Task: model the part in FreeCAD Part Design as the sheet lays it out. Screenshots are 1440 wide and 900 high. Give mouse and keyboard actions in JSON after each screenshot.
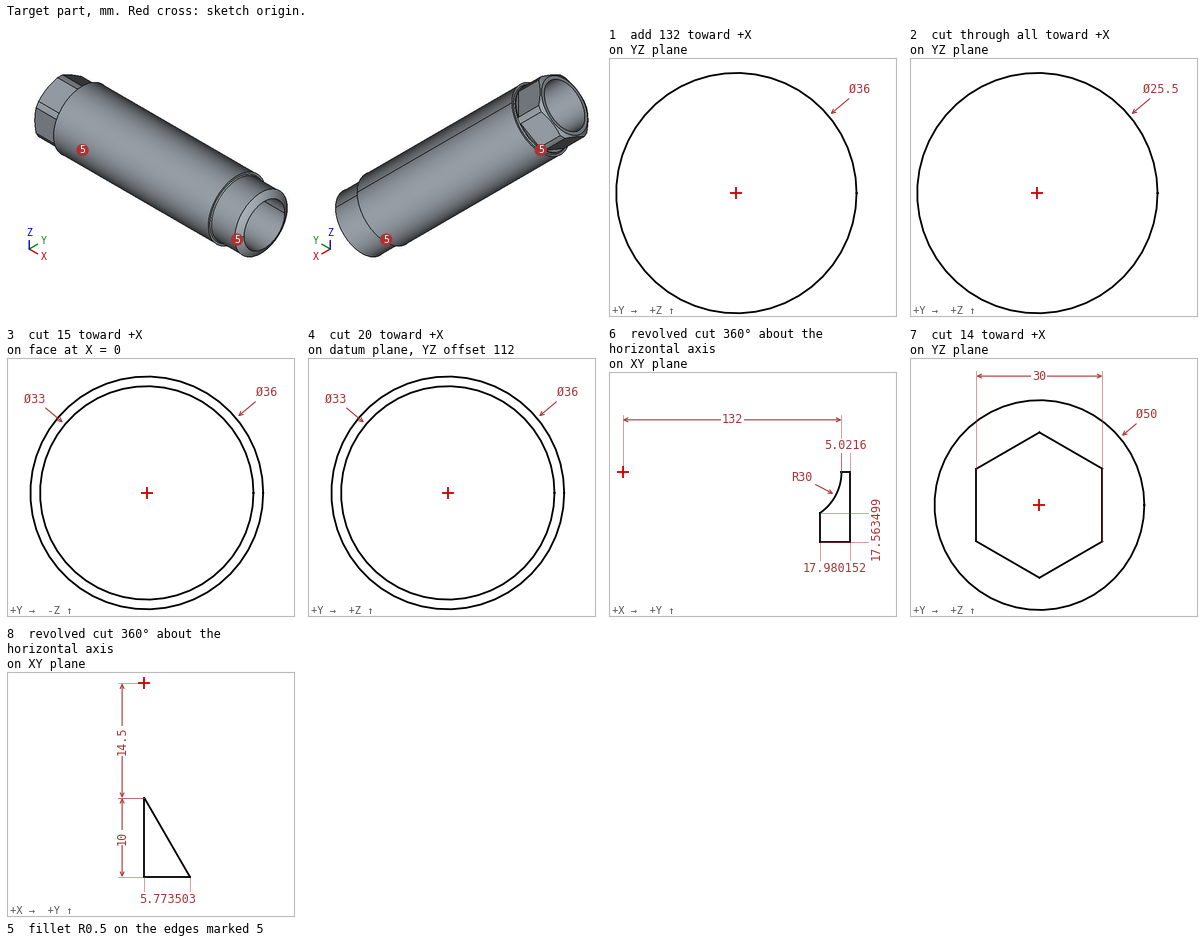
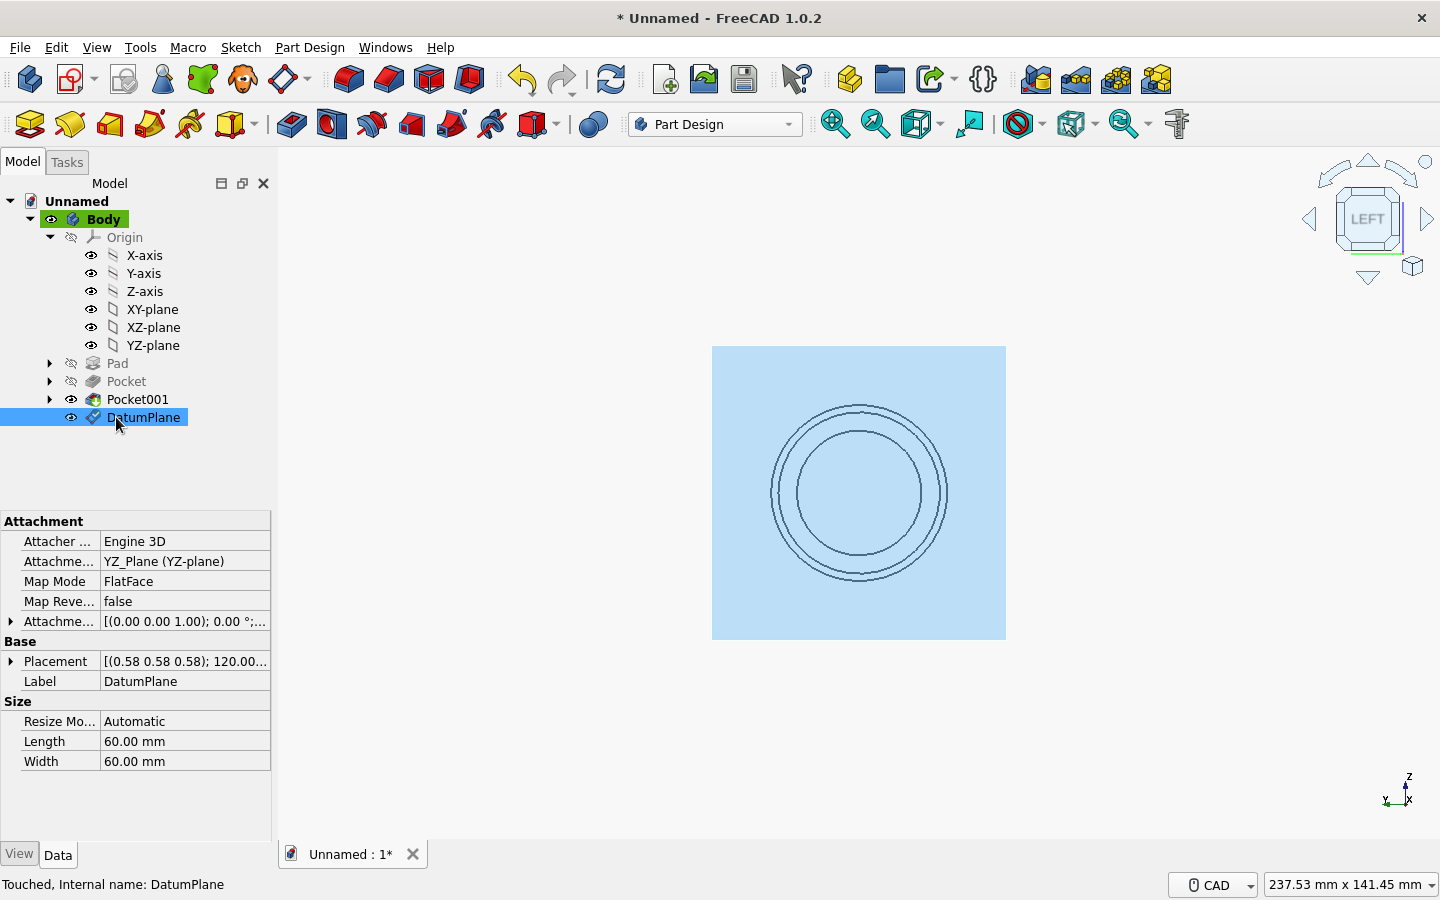
{"action": "left_click", "coordinate": [70, 80]}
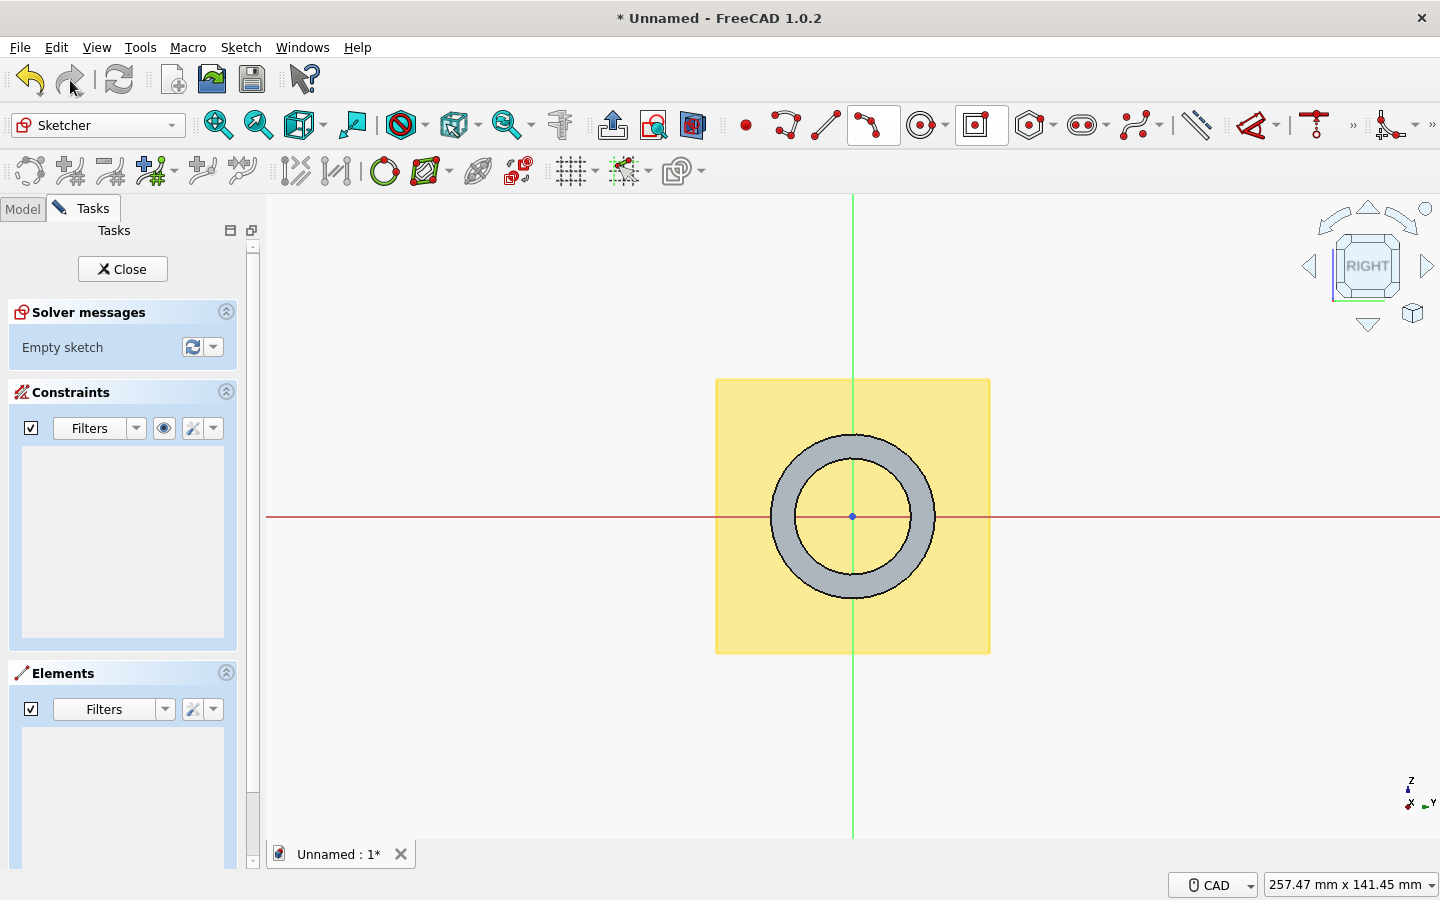
{"action": "key", "text": "q s"}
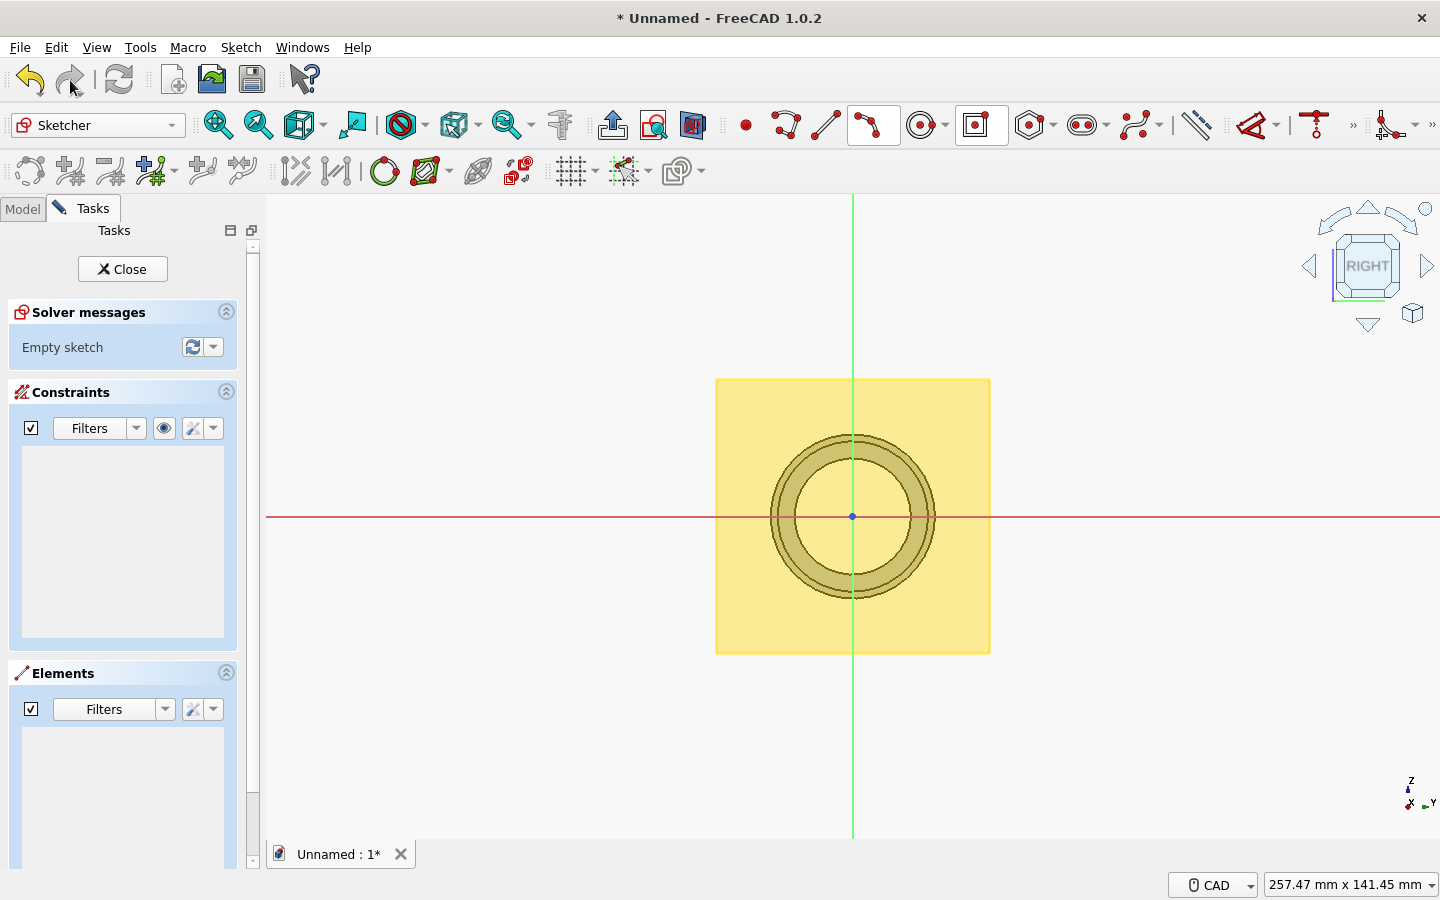
{"action": "scroll", "coordinate": [893, 516], "scroll_direction": "up", "scroll_amount": 5}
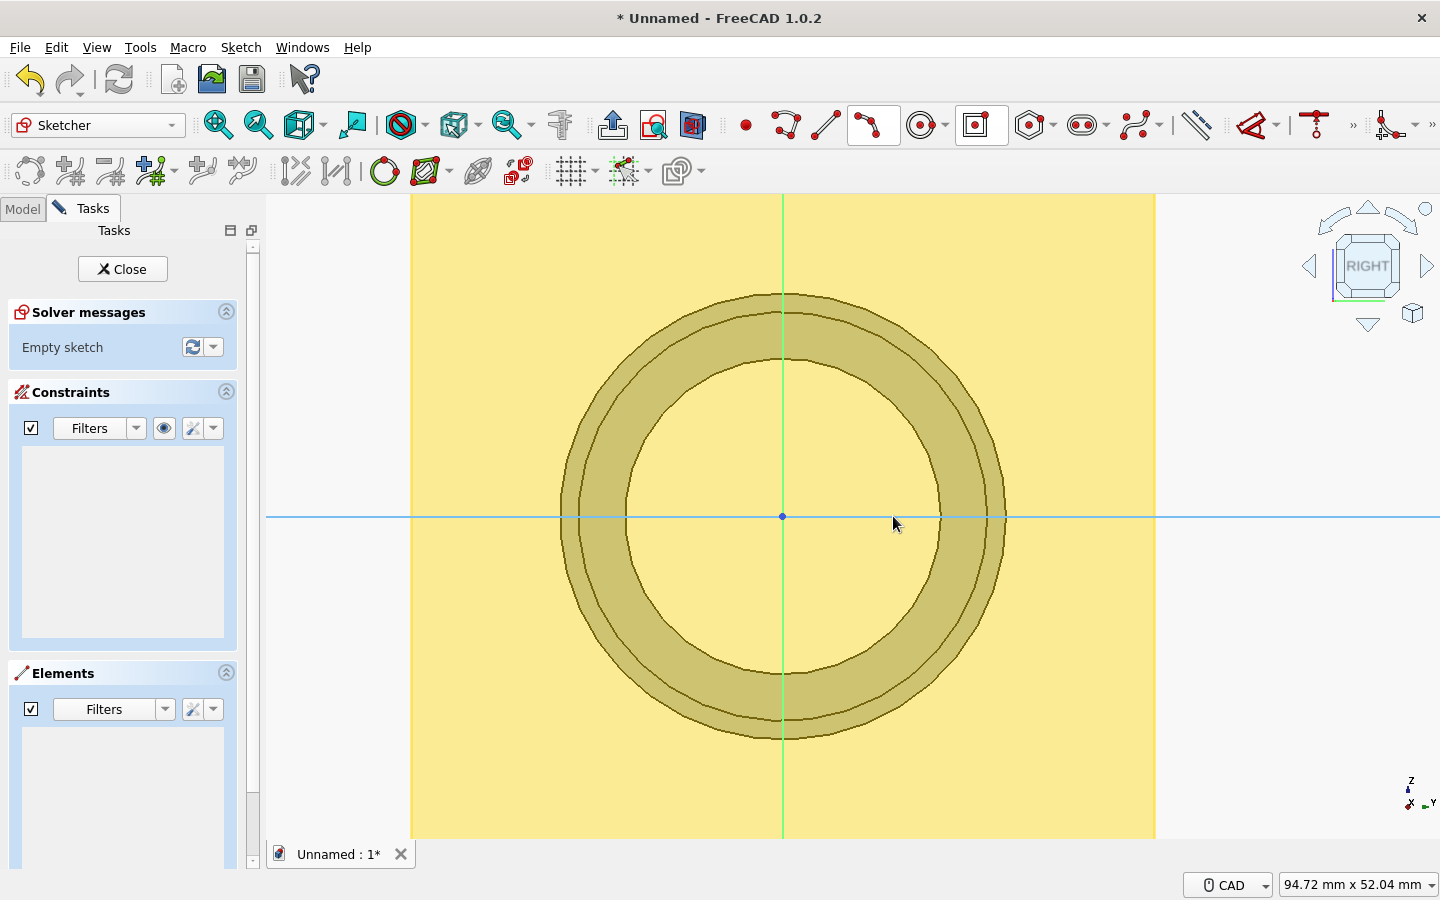
{"action": "left_click", "coordinate": [922, 126]}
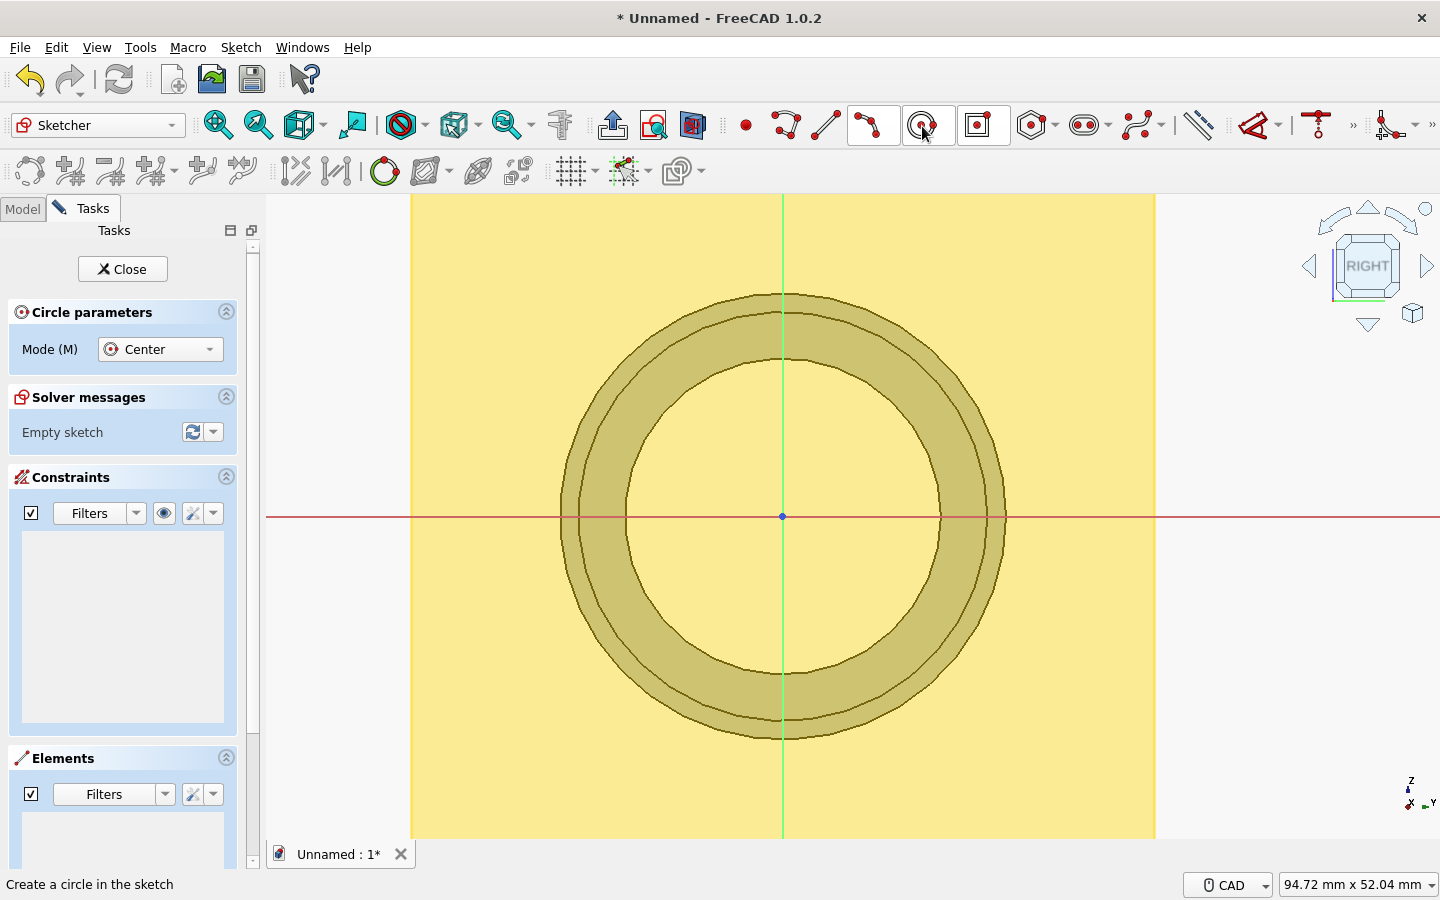
{"action": "left_click", "coordinate": [783, 516]}
{"action": "mouse_move", "coordinate": [941, 359]}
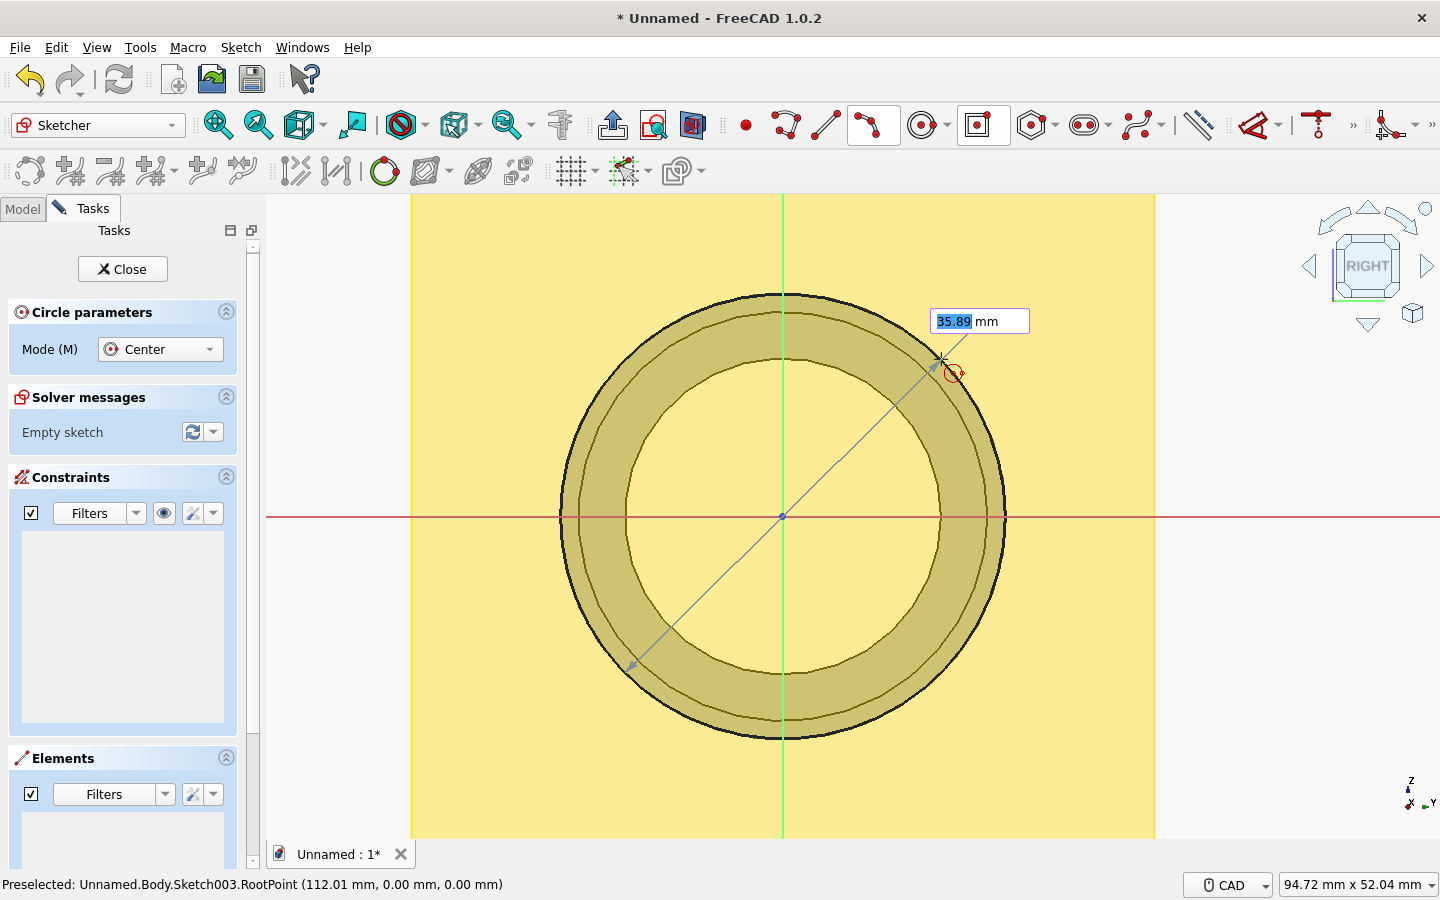
{"action": "type", "text": "36"}
{"action": "key", "text": "Return"}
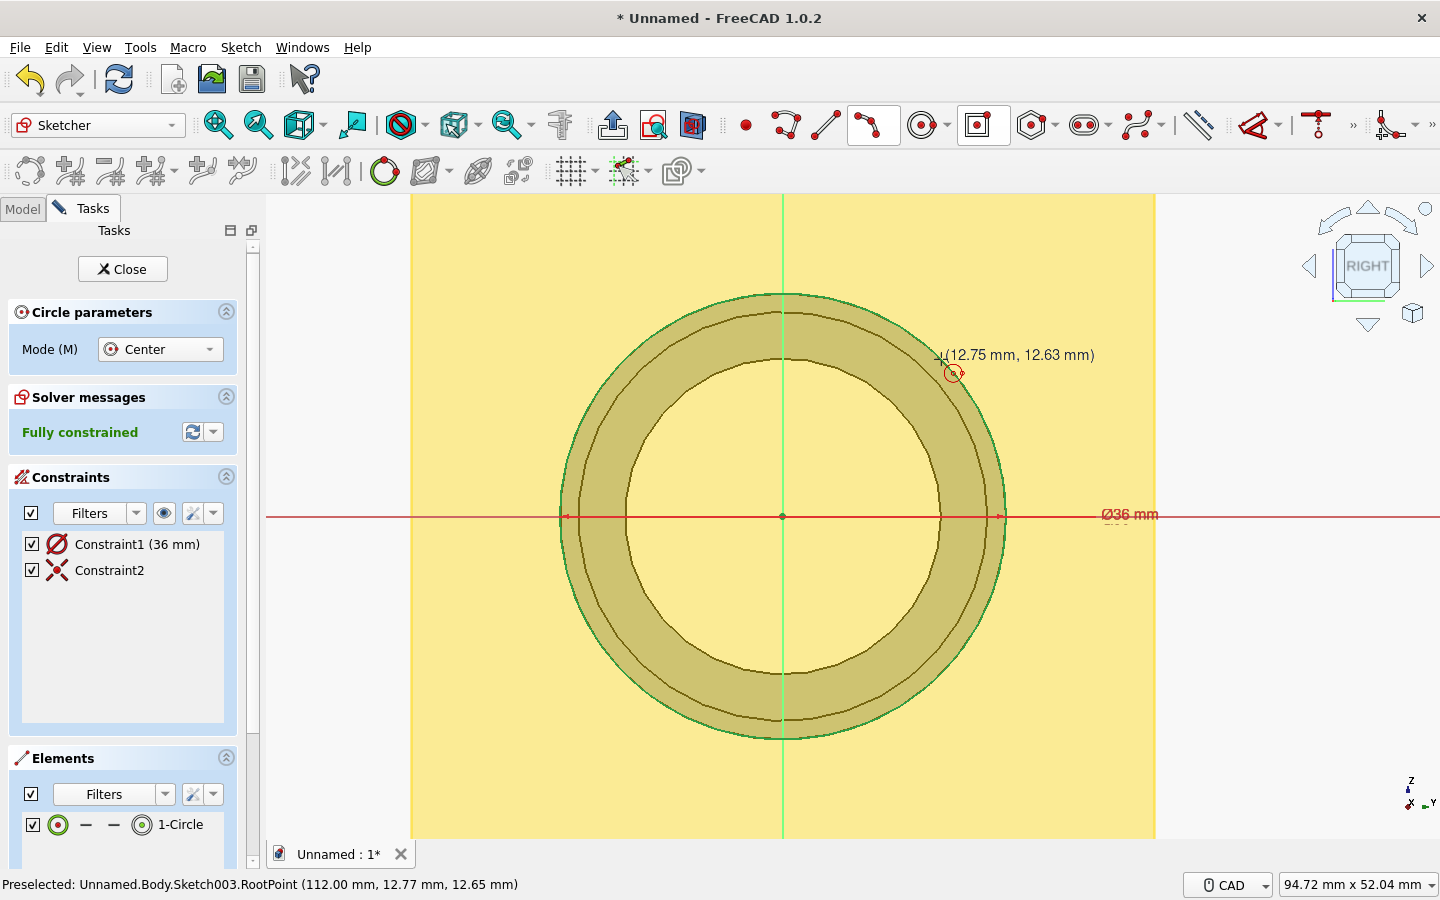
{"action": "left_click", "coordinate": [783, 516]}
{"action": "mouse_move", "coordinate": [928, 372]}